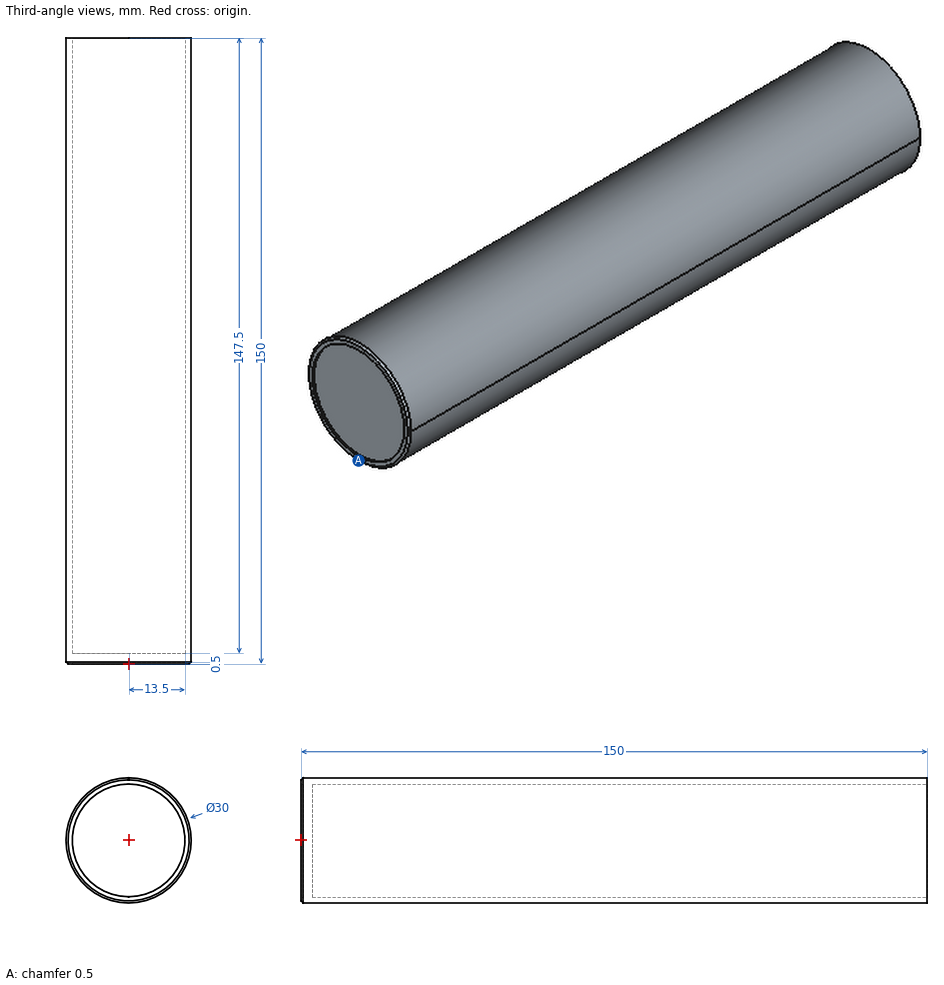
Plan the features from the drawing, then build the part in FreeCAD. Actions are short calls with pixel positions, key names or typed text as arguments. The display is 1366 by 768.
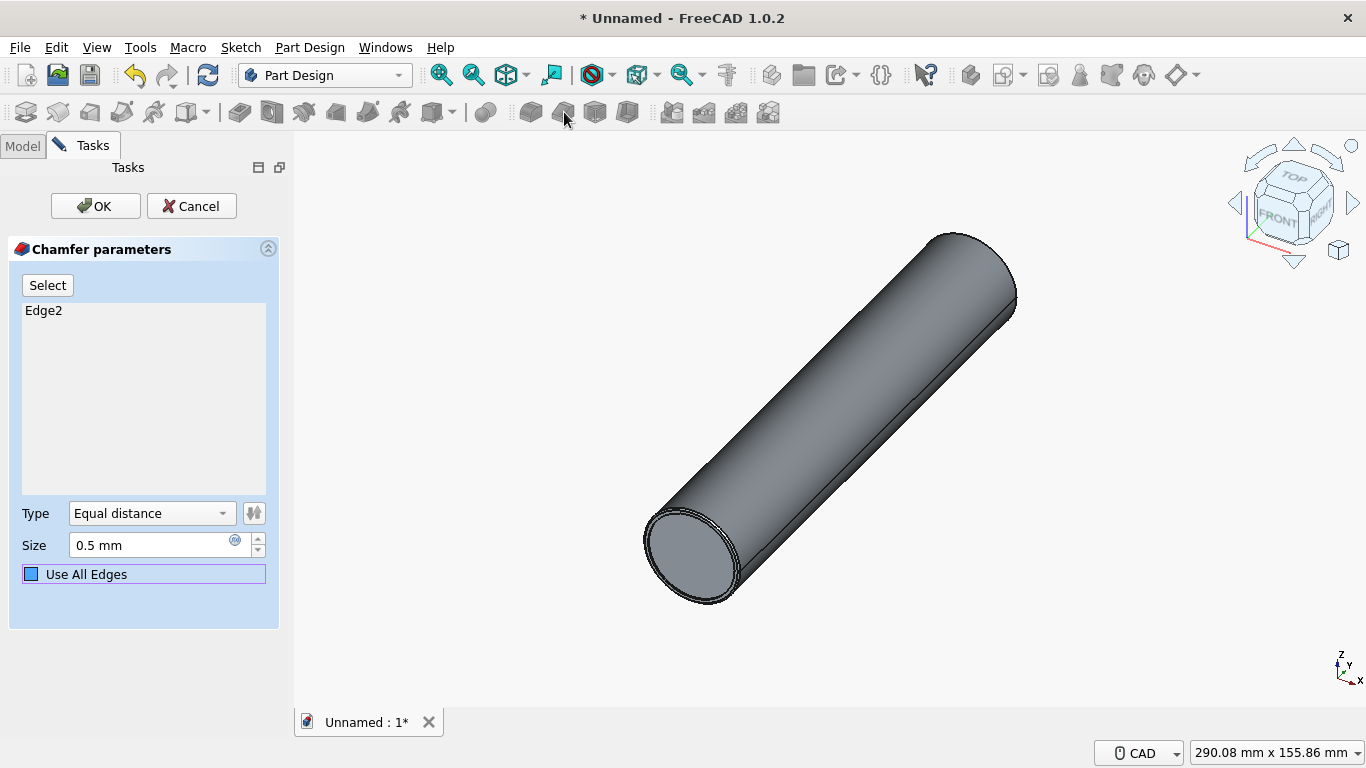
click(96, 206)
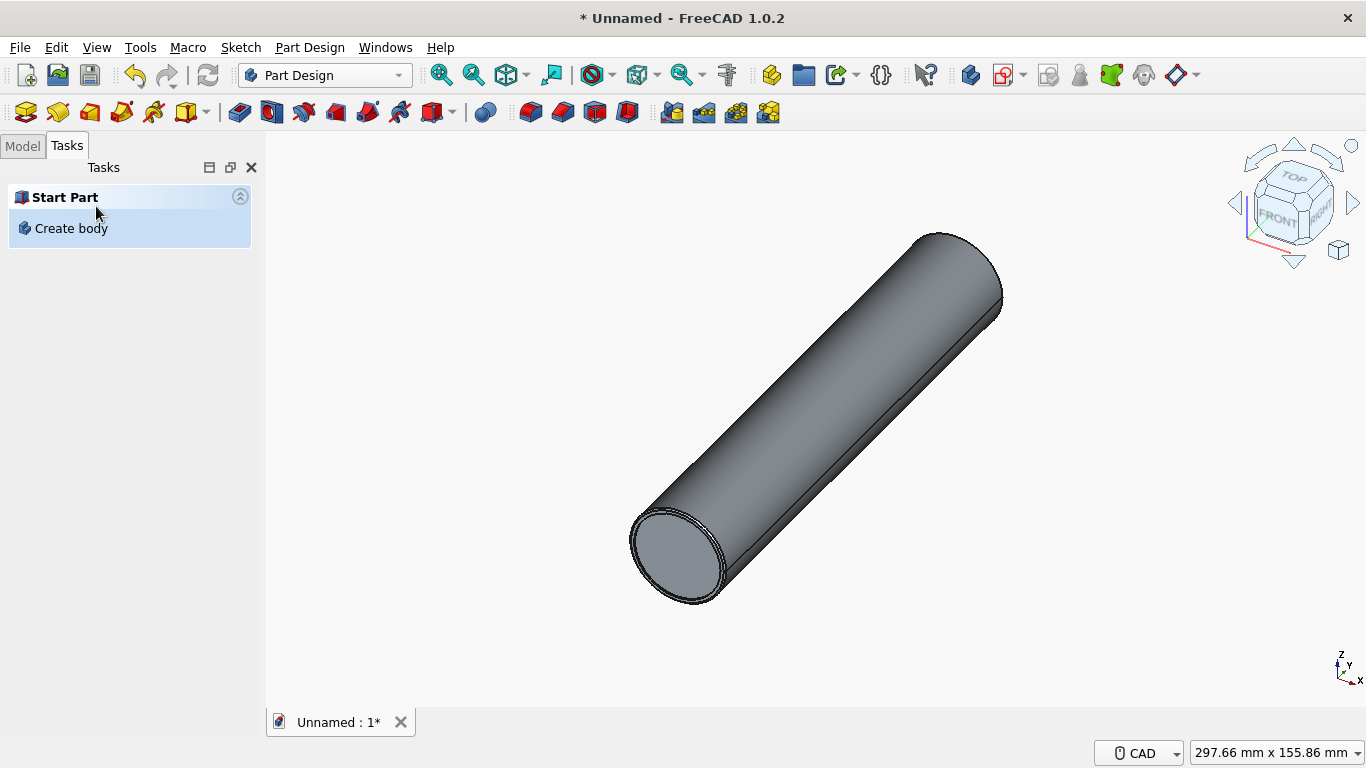
key(0)